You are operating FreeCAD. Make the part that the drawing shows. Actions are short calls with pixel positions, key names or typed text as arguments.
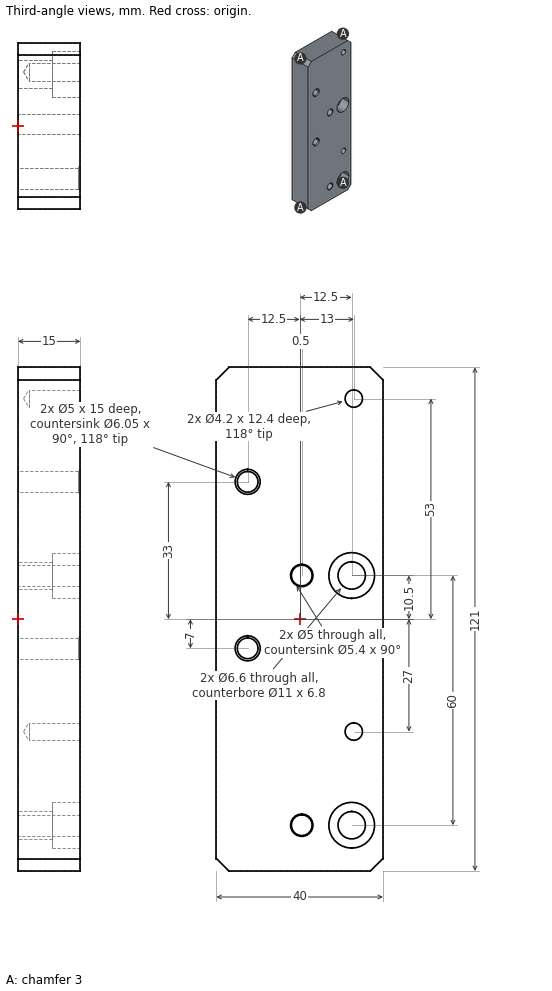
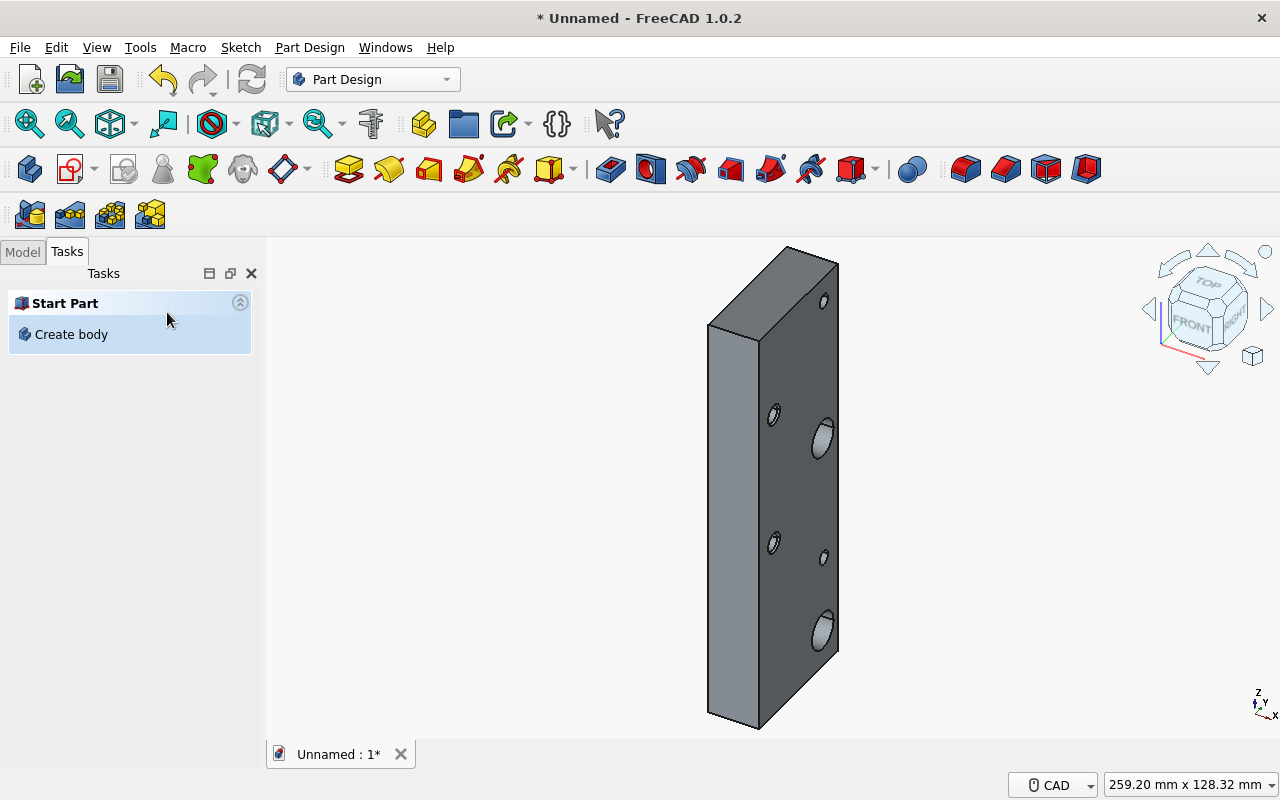
click(787, 617)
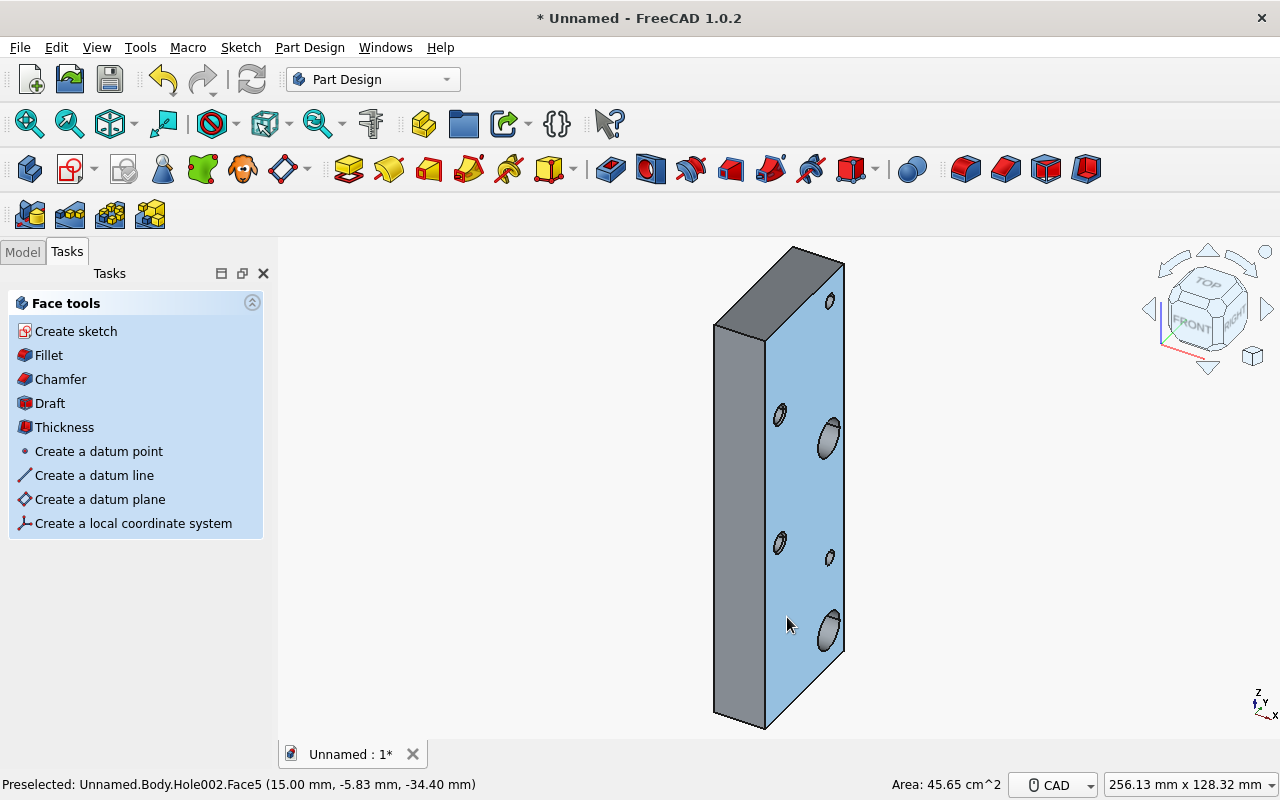
click(70, 170)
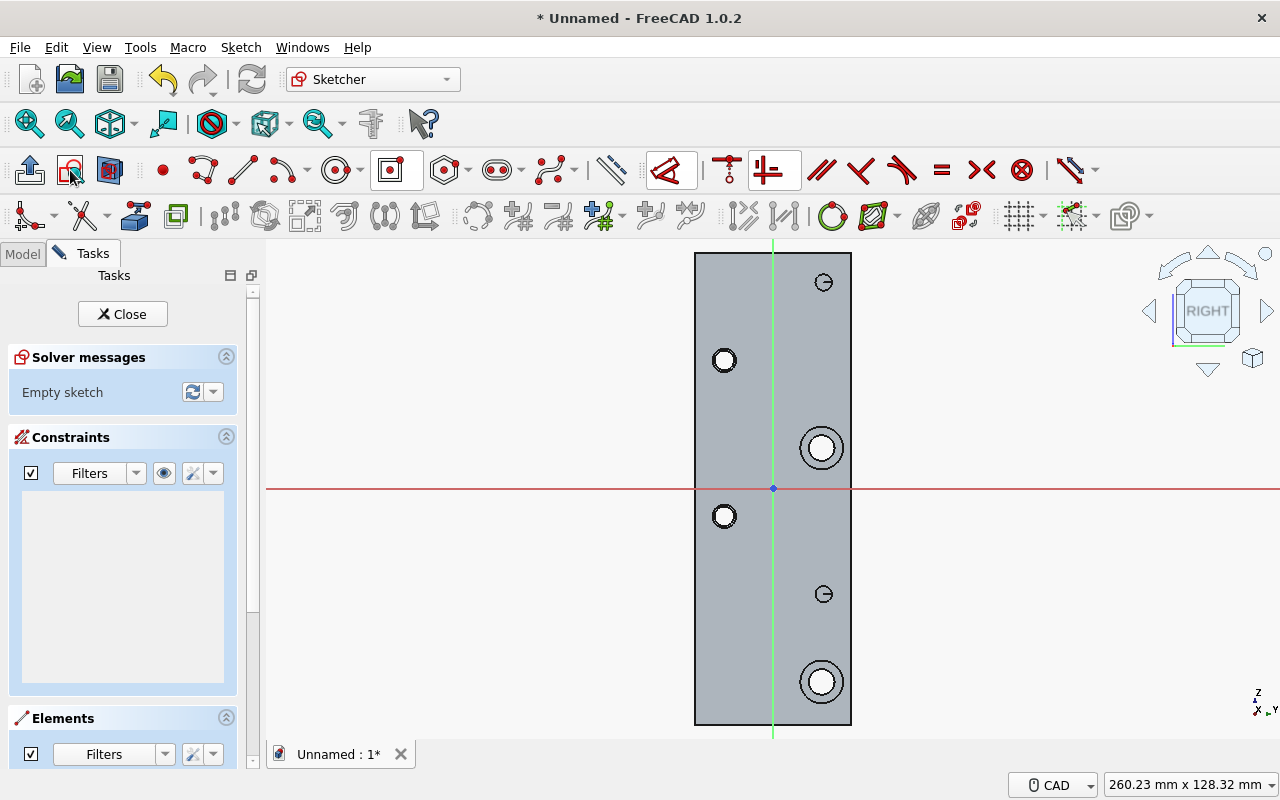
scroll(386, 267, down, 1)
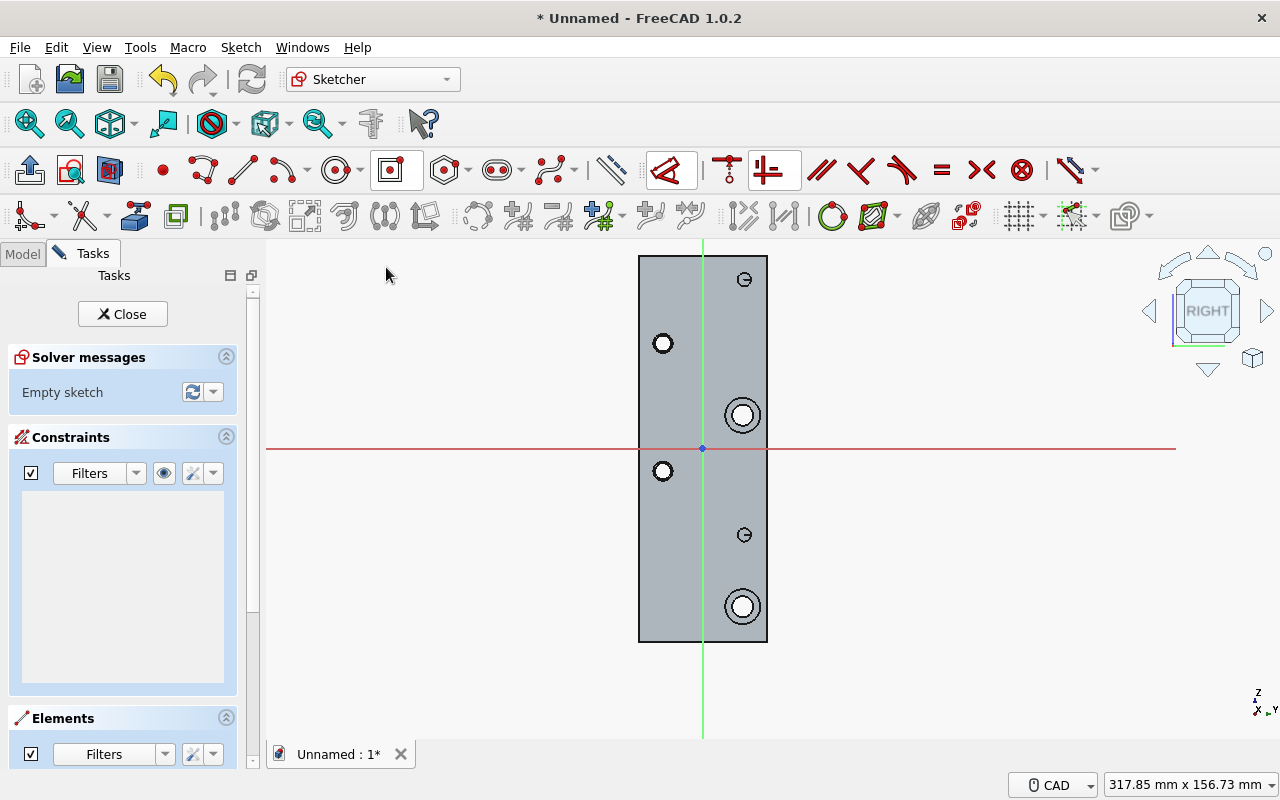
scroll(704, 556, up, 2)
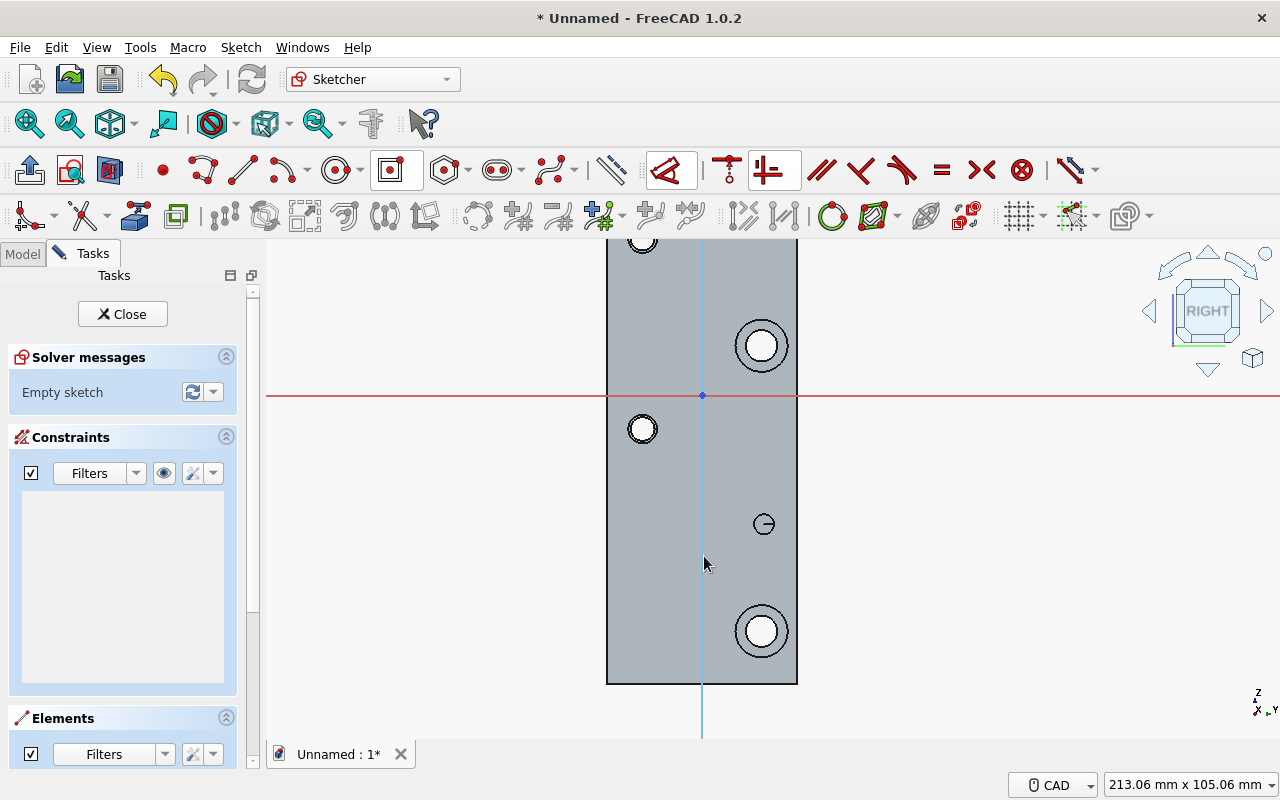
click(336, 170)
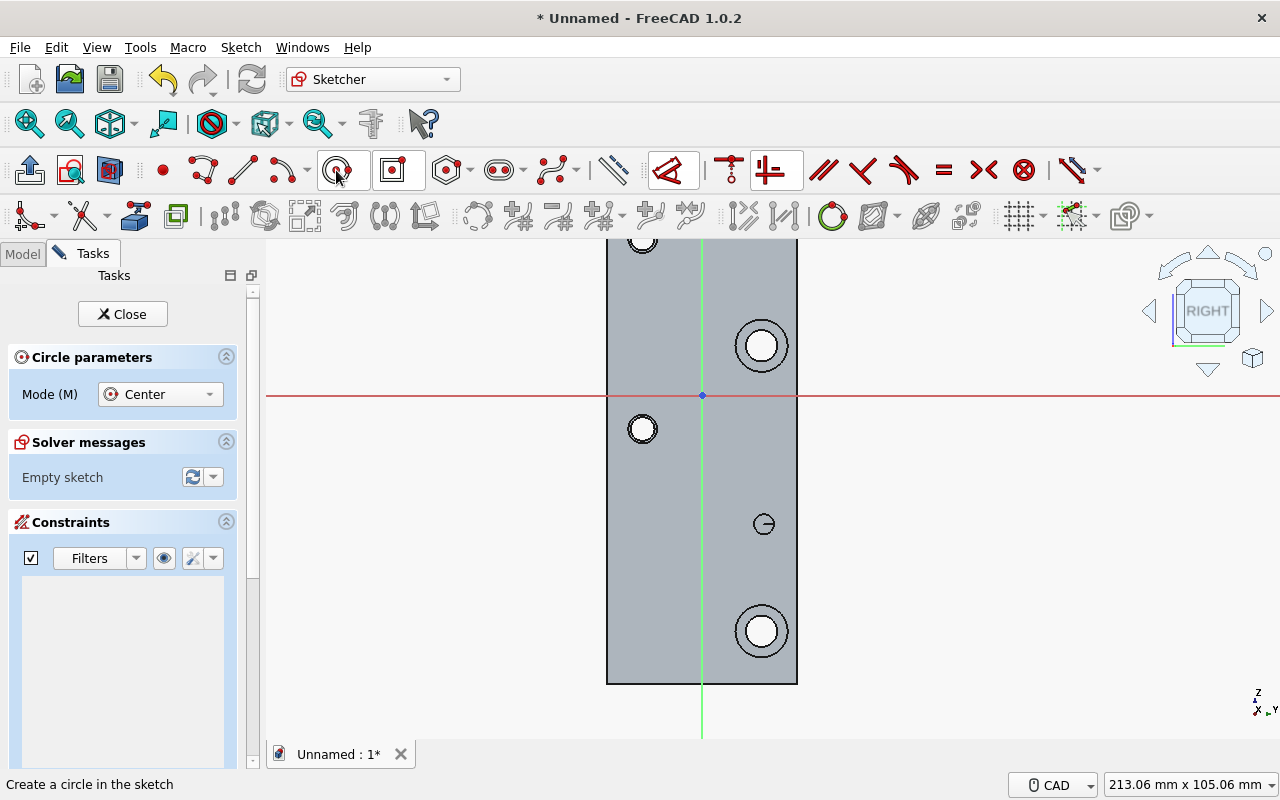
scroll(704, 346, up, 10)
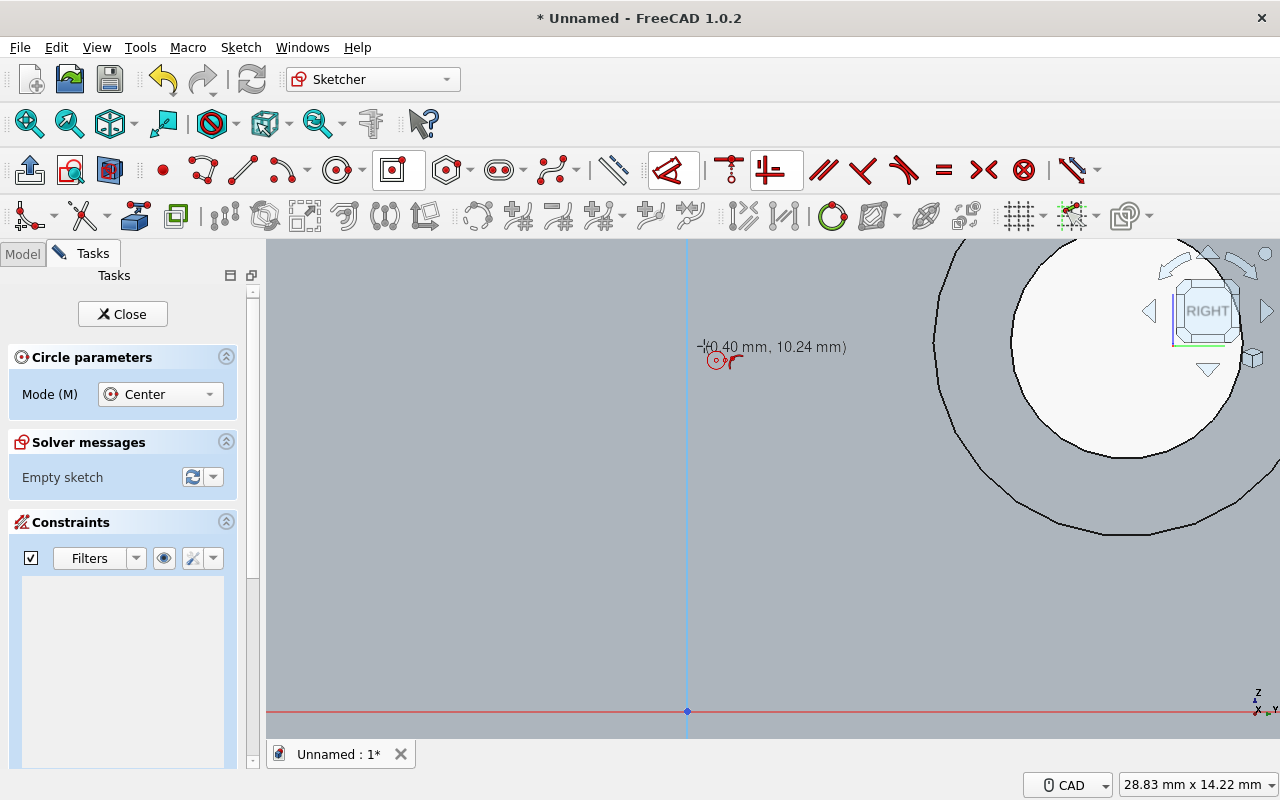
click(705, 343)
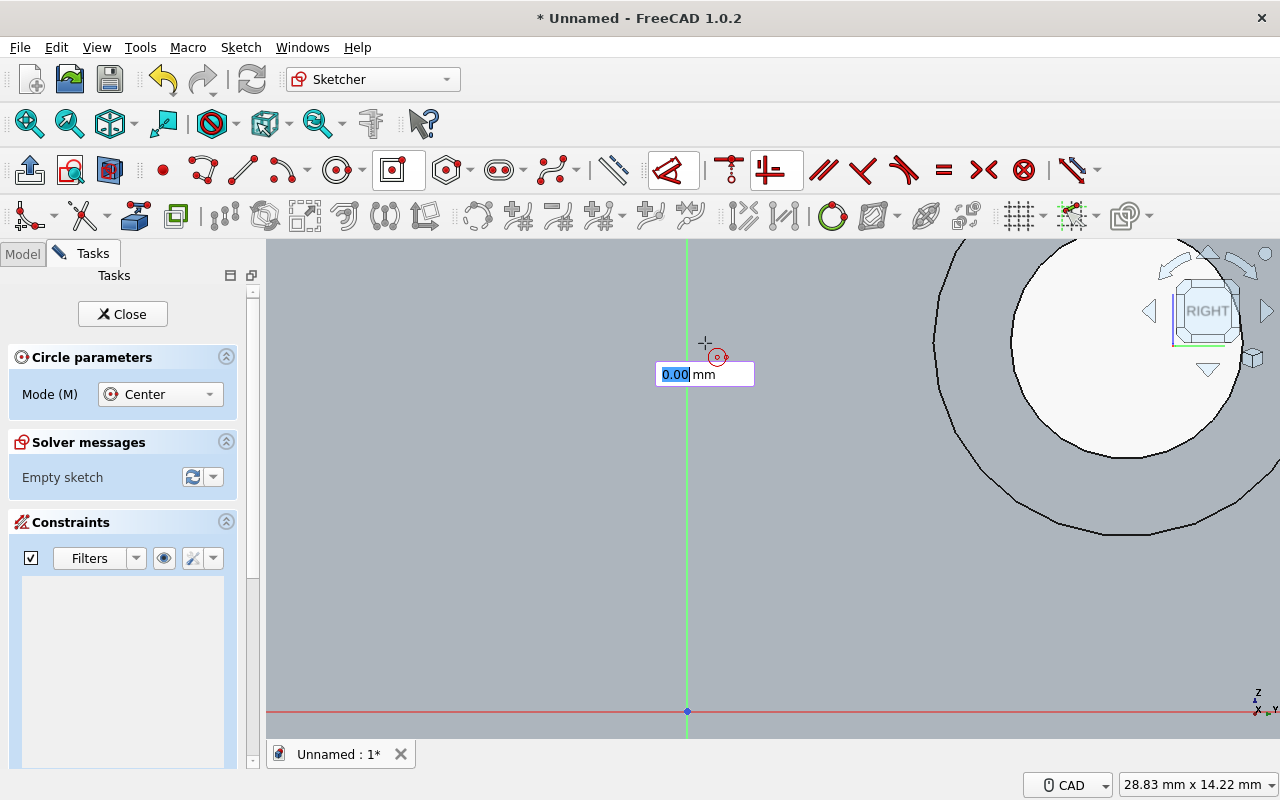
scroll(704, 347, down, 10)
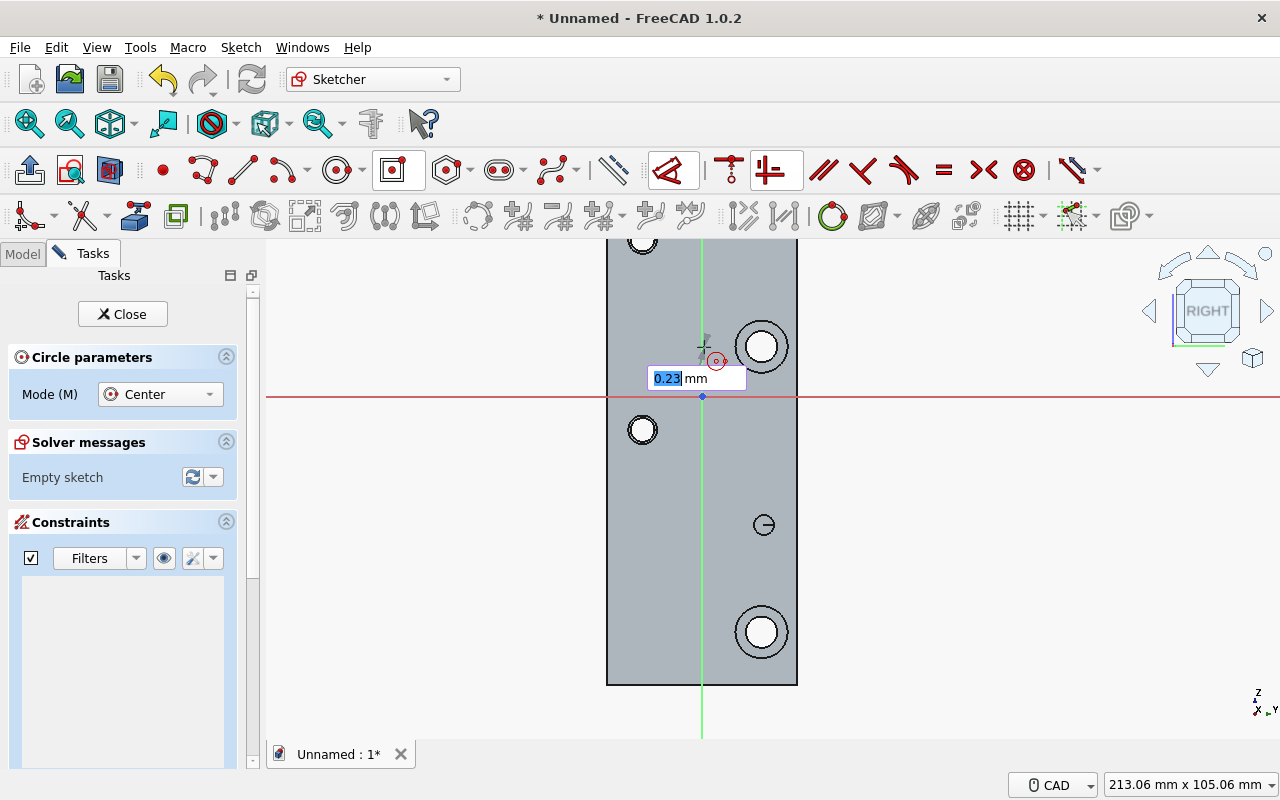
scroll(713, 338, up, 2)
move(713, 338)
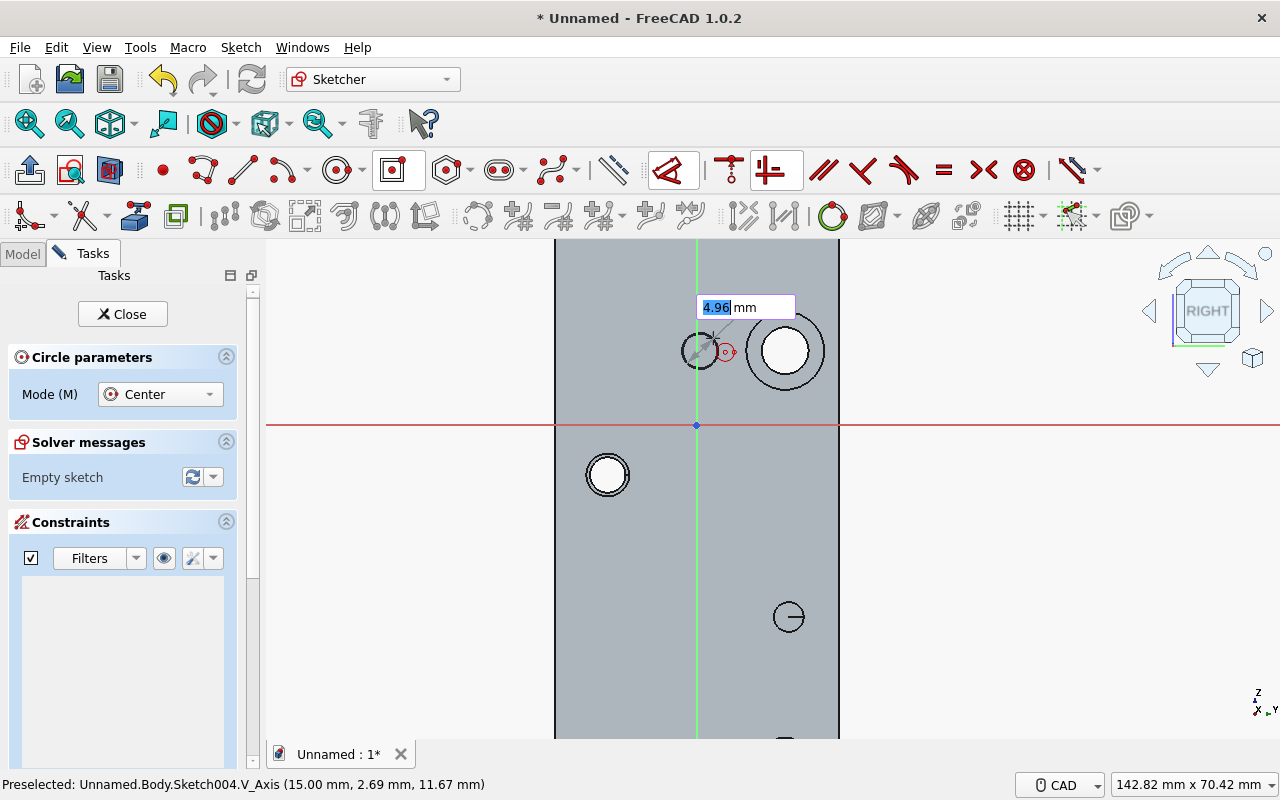
text(5)
key(Return)